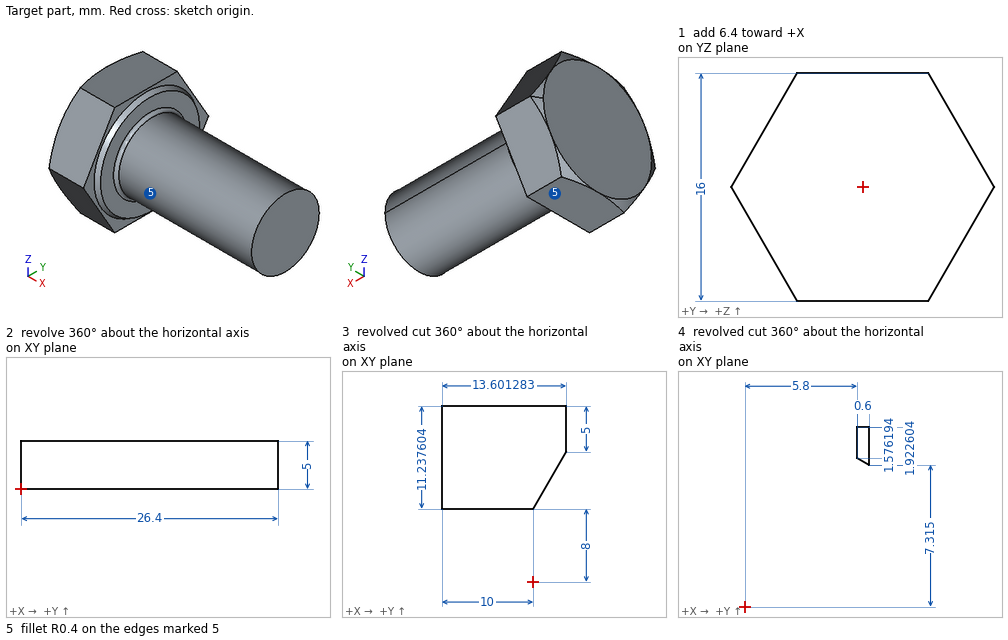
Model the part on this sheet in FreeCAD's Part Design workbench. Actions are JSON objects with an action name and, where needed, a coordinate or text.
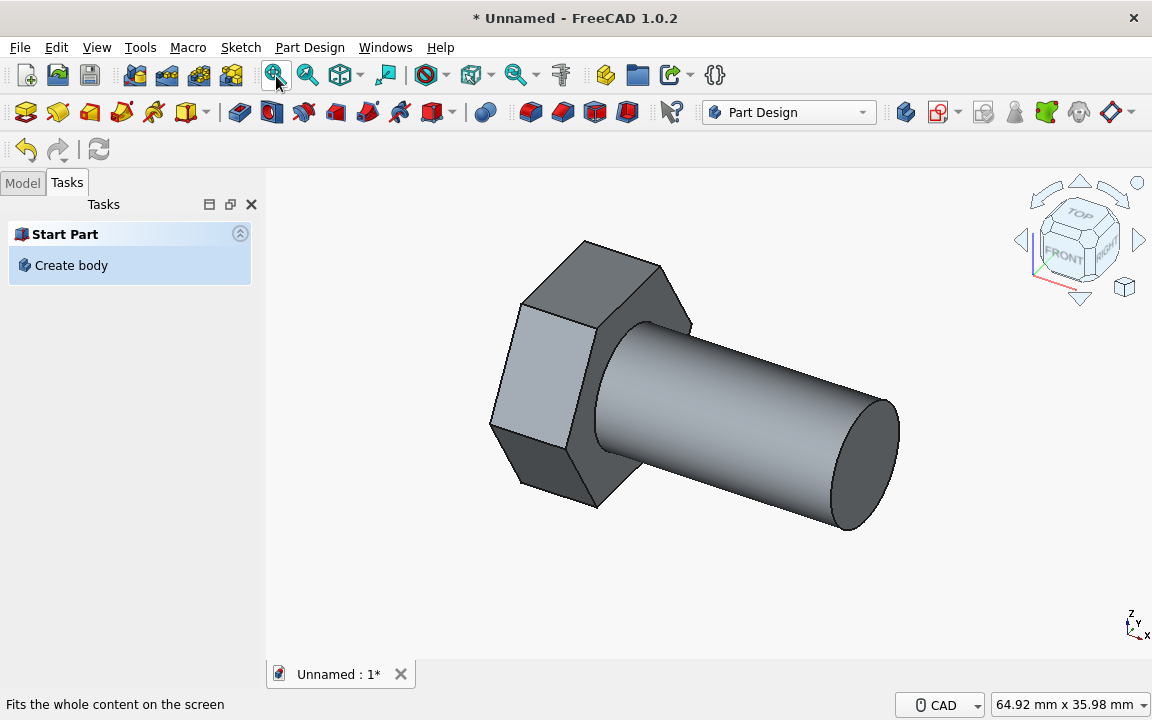
{"action": "left_click", "coordinate": [938, 112]}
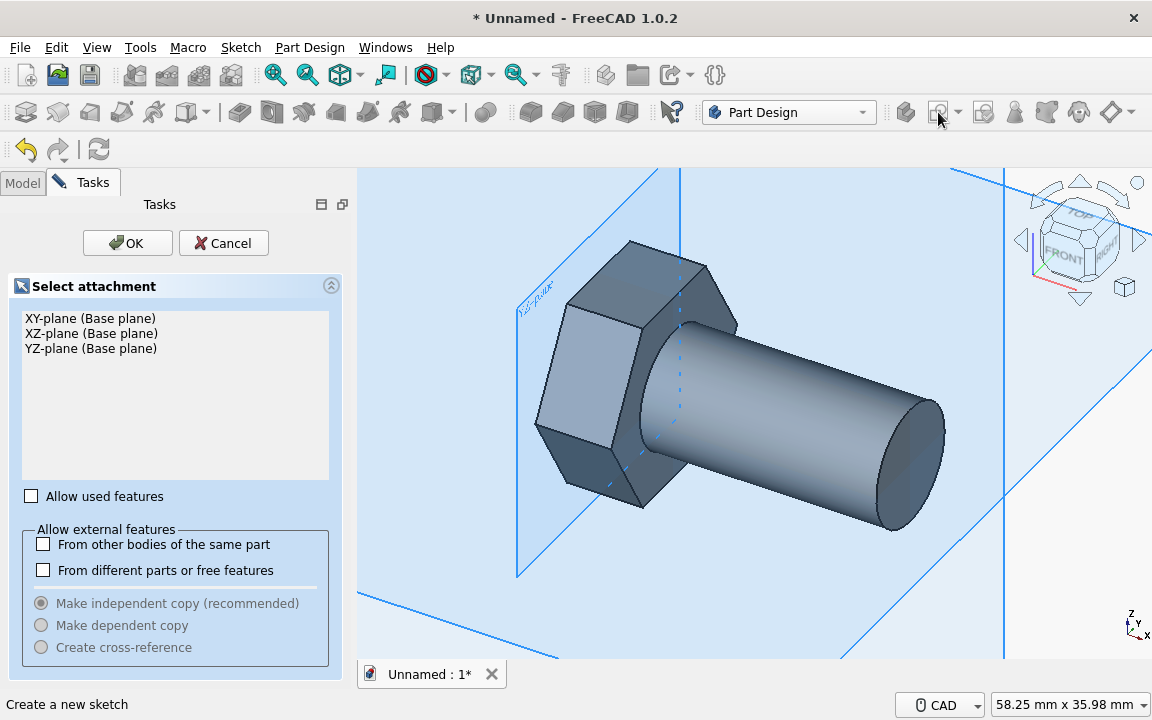
{"action": "left_click", "coordinate": [82, 318]}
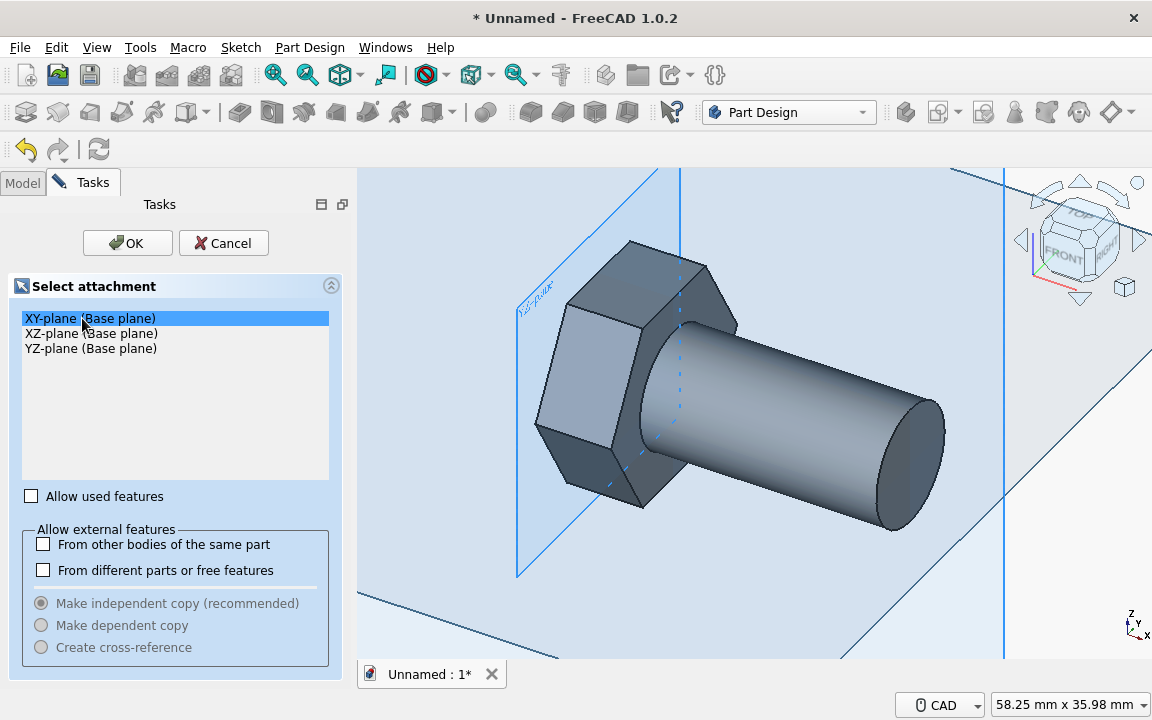
{"action": "left_click", "coordinate": [128, 243]}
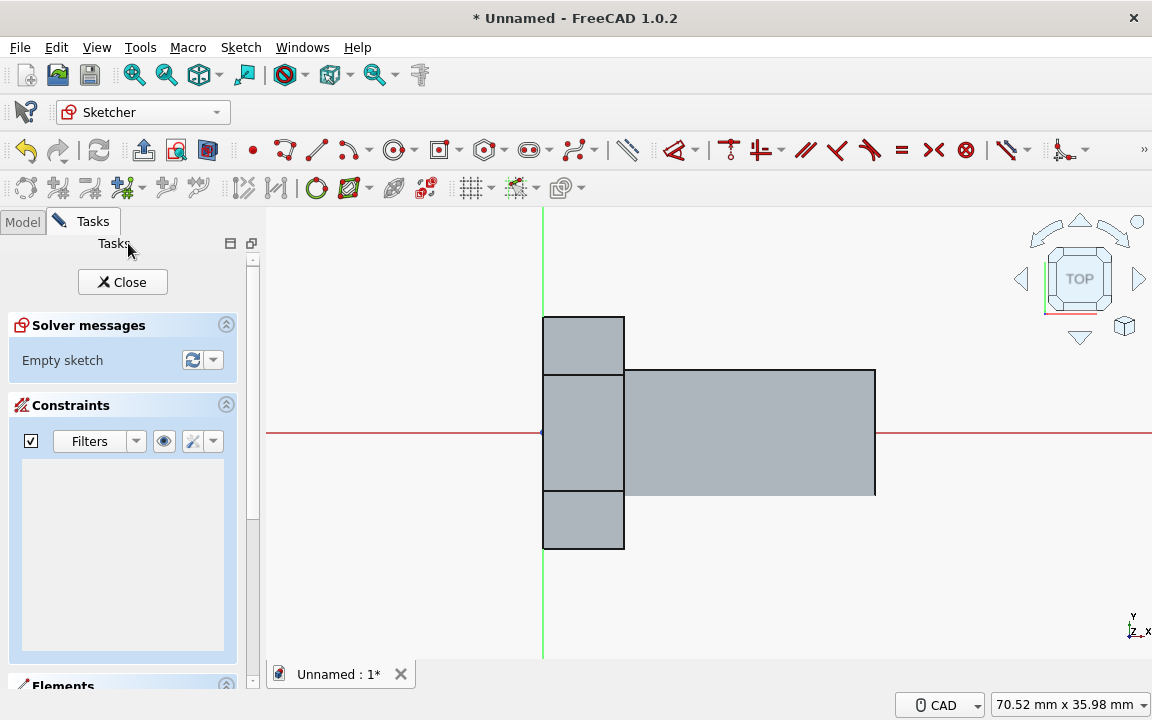
{"action": "left_click", "coordinate": [208, 150]}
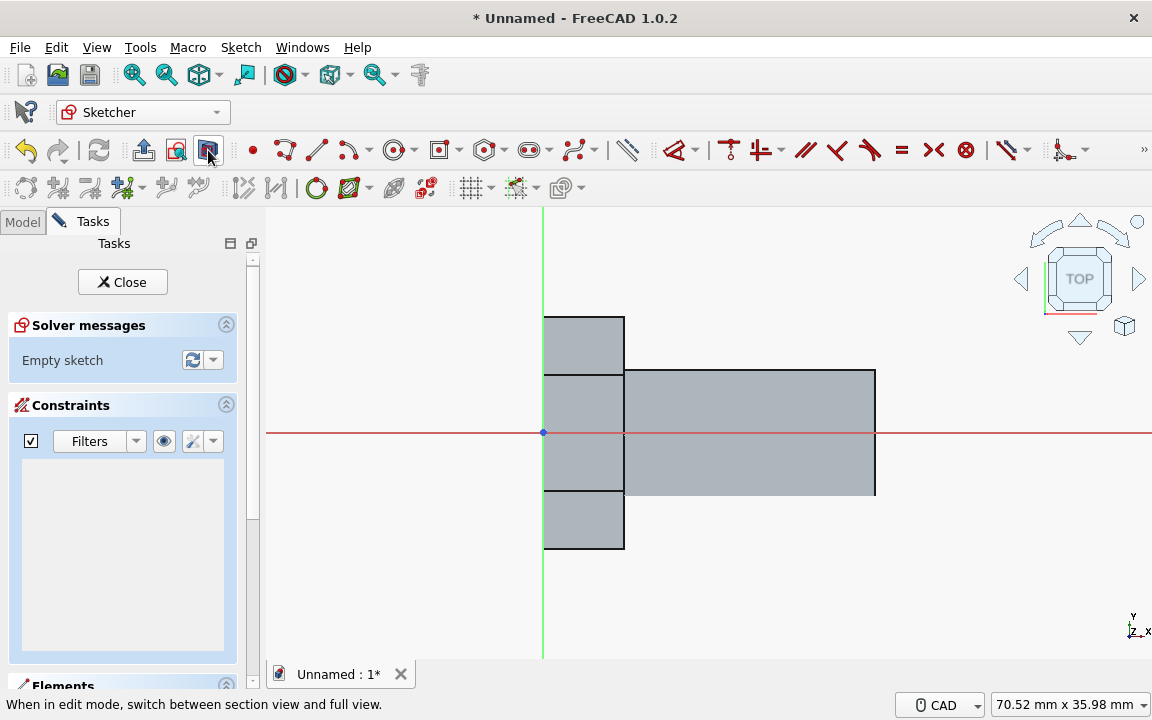
{"action": "scroll", "coordinate": [987, 631], "scroll_direction": "down", "scroll_amount": 1}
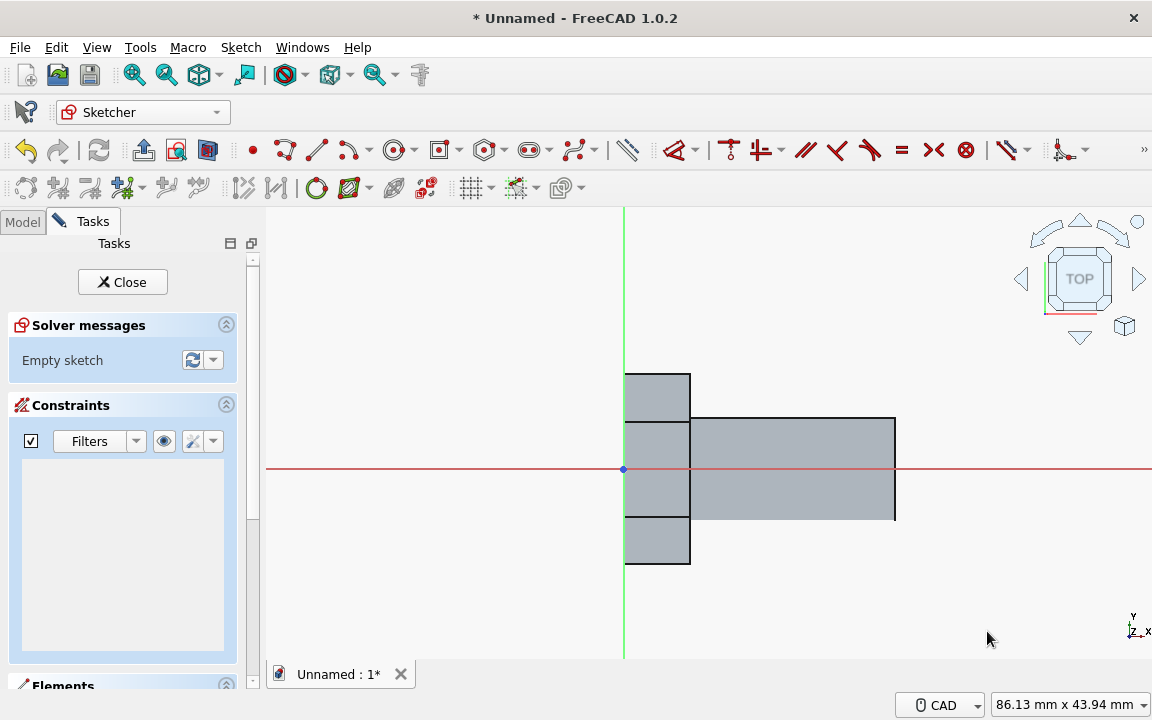
{"action": "scroll", "coordinate": [490, 242], "scroll_direction": "up", "scroll_amount": 2}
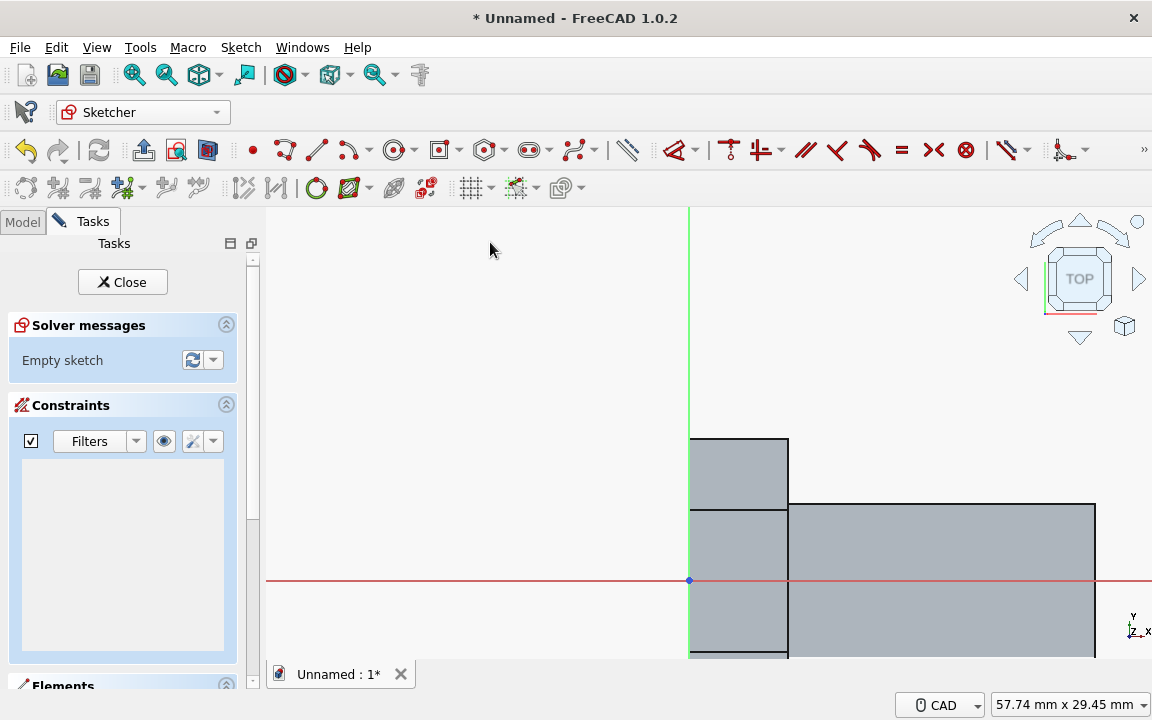
{"action": "left_click", "coordinate": [286, 150]}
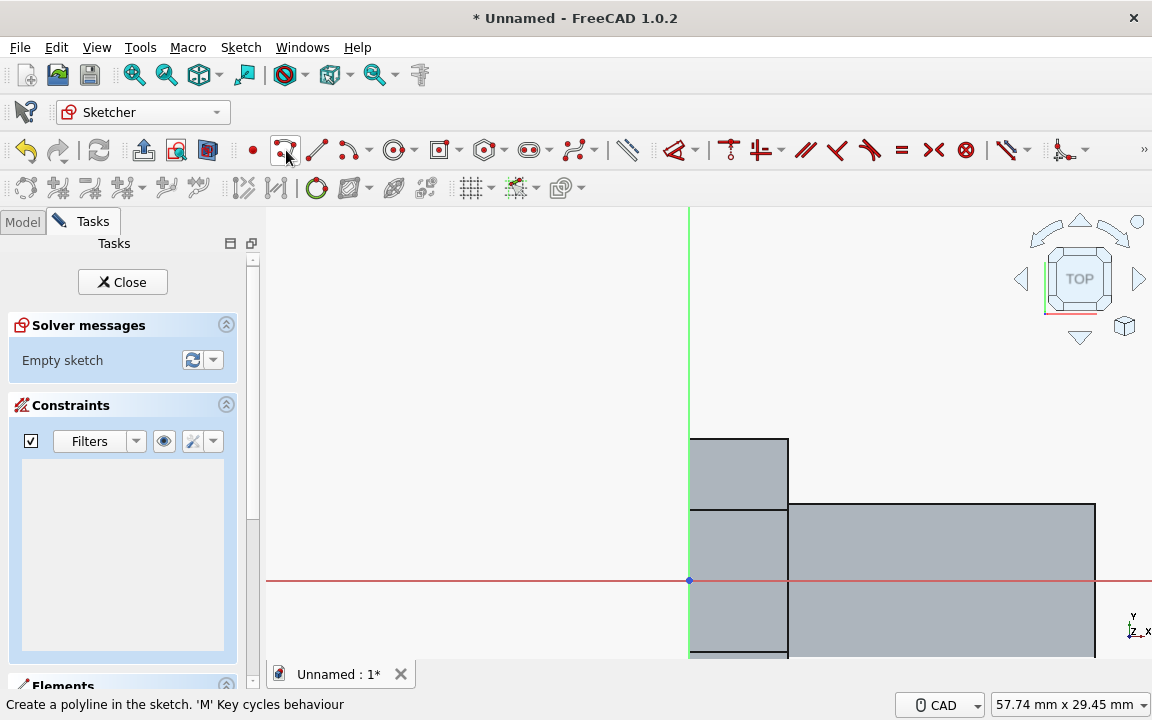
{"action": "left_click", "coordinate": [689, 458]}
{"action": "left_click", "coordinate": [745, 362]}
{"action": "left_click", "coordinate": [745, 285]}
{"action": "left_click", "coordinate": [536, 285]}
{"action": "left_click", "coordinate": [536, 458]}
{"action": "left_click", "coordinate": [689, 459]}
{"action": "key", "text": "Escape"}
{"action": "key", "text": "Escape"}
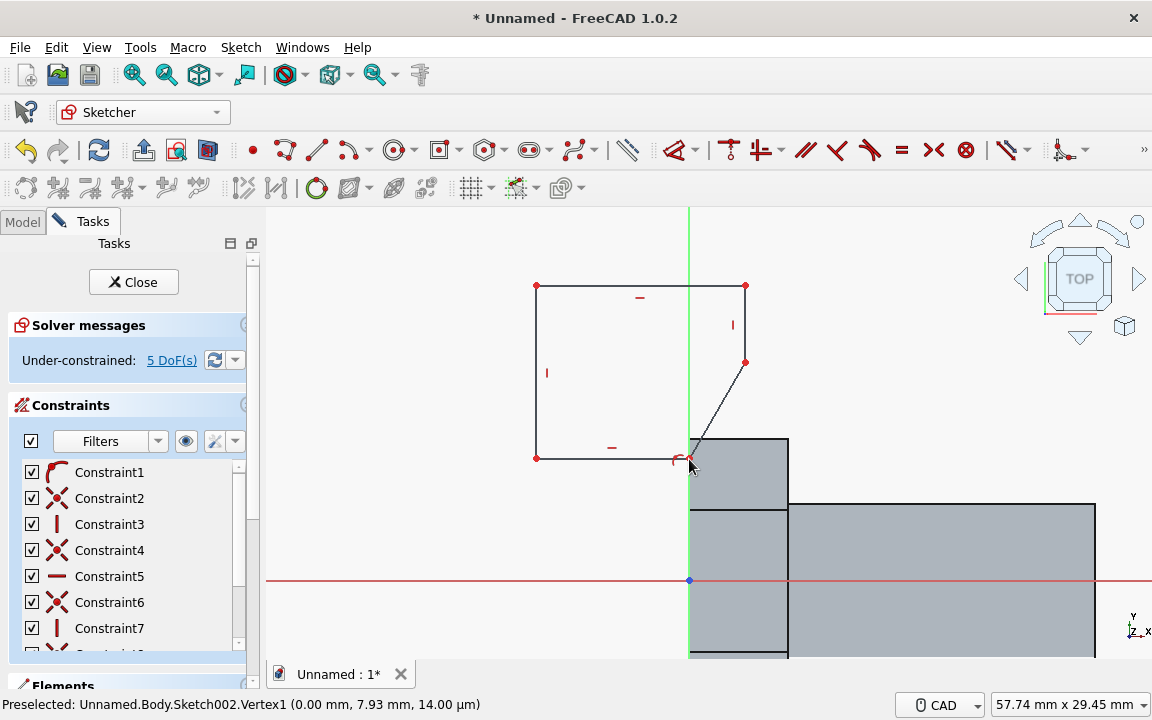
{"action": "left_click", "coordinate": [674, 150]}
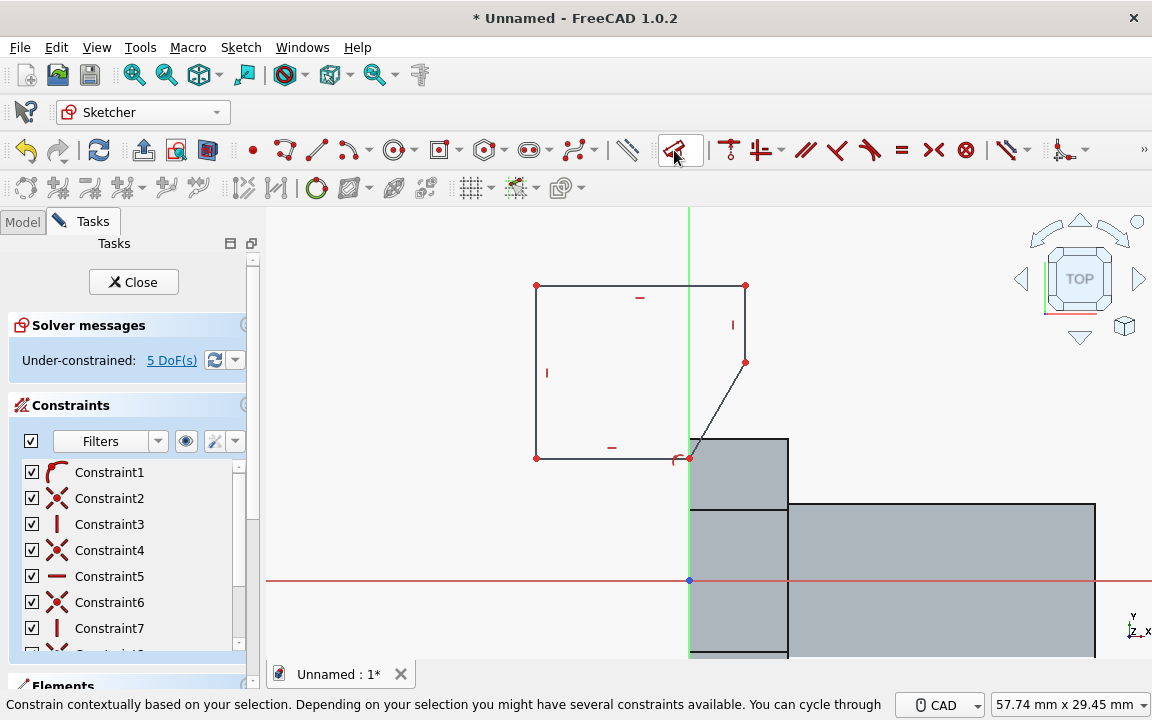
{"action": "left_click", "coordinate": [745, 340]}
{"action": "left_click", "coordinate": [779, 325]}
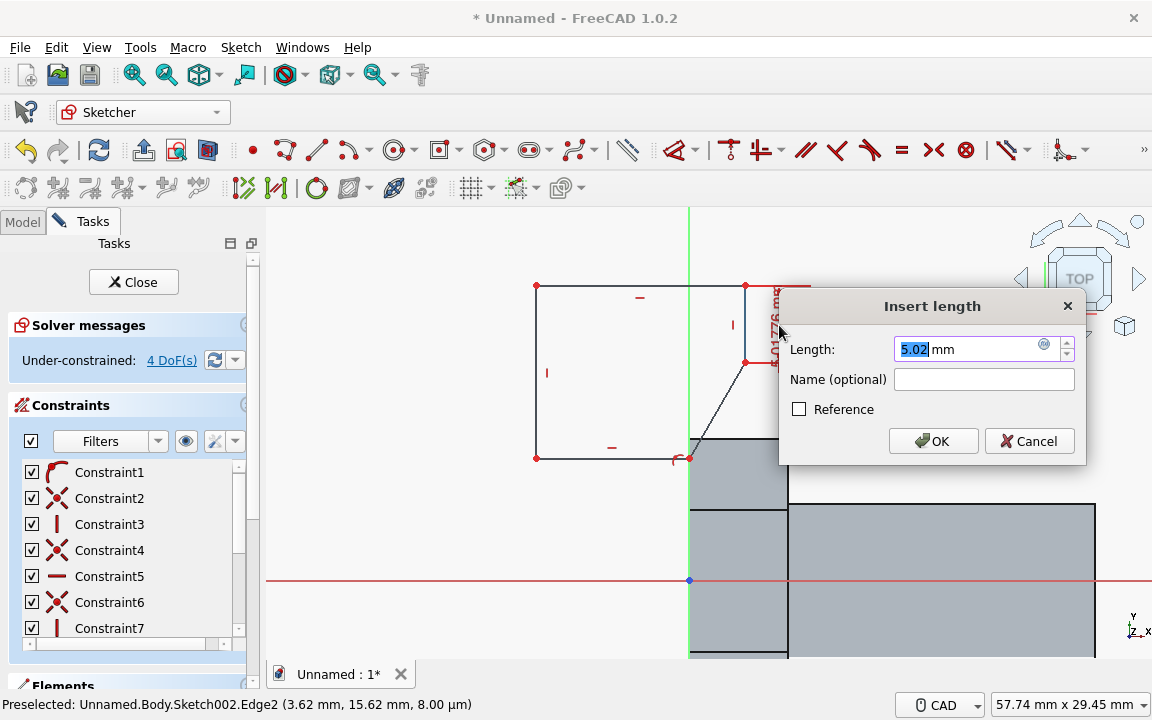
{"action": "type", "text": "5"}
{"action": "key", "text": "Return"}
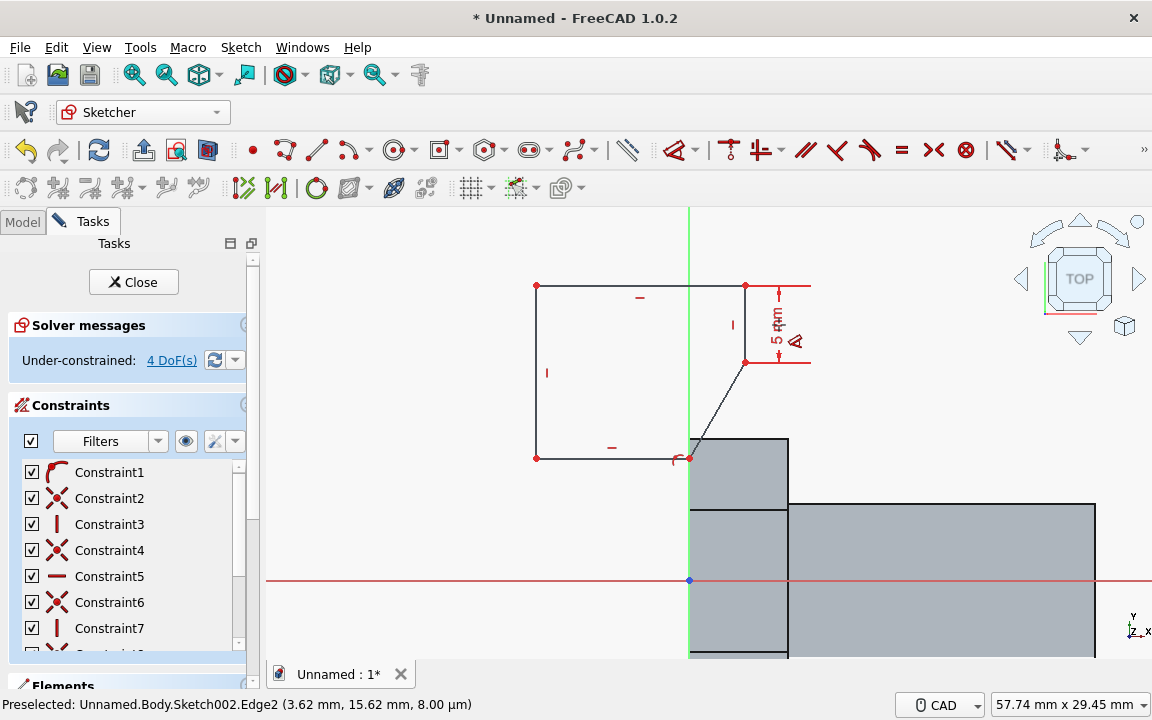
{"action": "left_click", "coordinate": [582, 459]}
{"action": "left_click", "coordinate": [613, 493]}